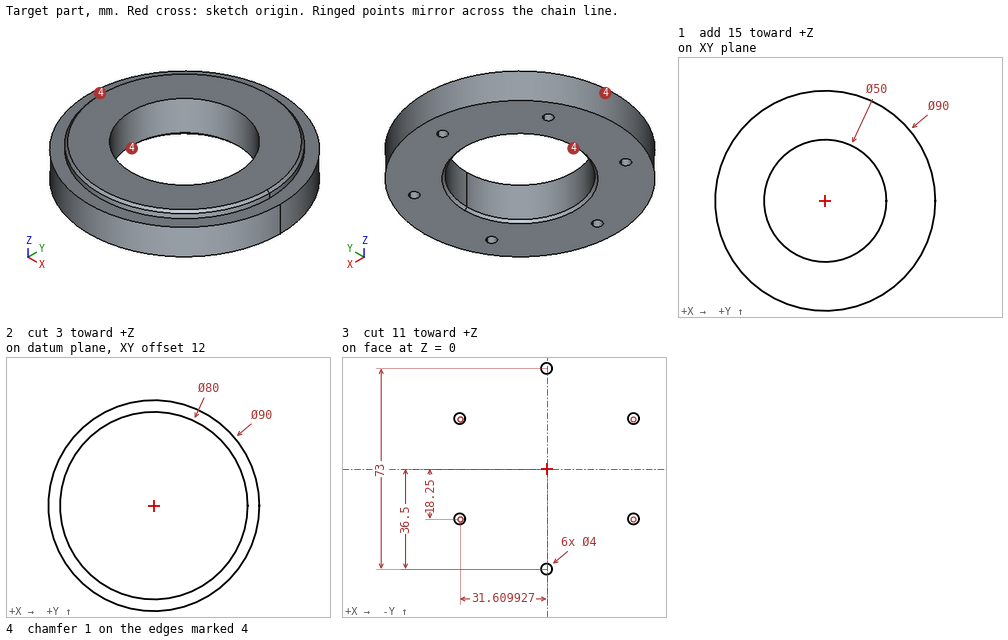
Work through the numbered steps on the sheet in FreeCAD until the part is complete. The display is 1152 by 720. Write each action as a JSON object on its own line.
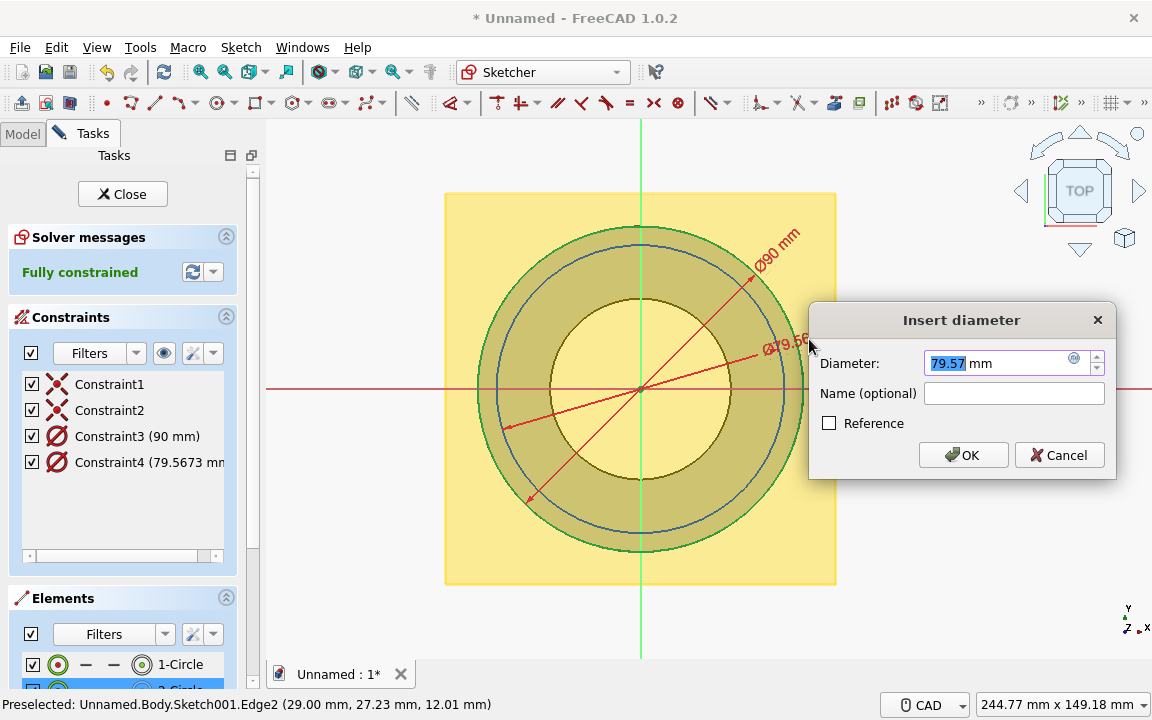
{"action": "type", "text": "80"}
{"action": "key", "text": "Return"}
{"action": "key", "text": "Escape"}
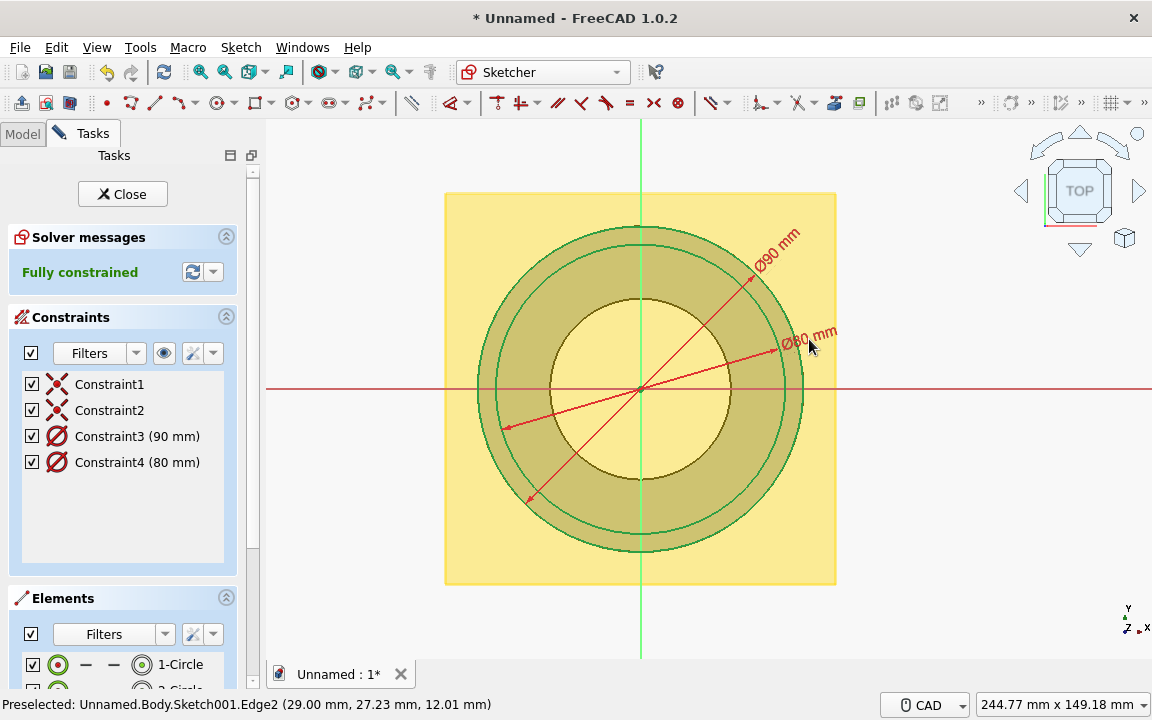
{"action": "left_click", "coordinate": [123, 194]}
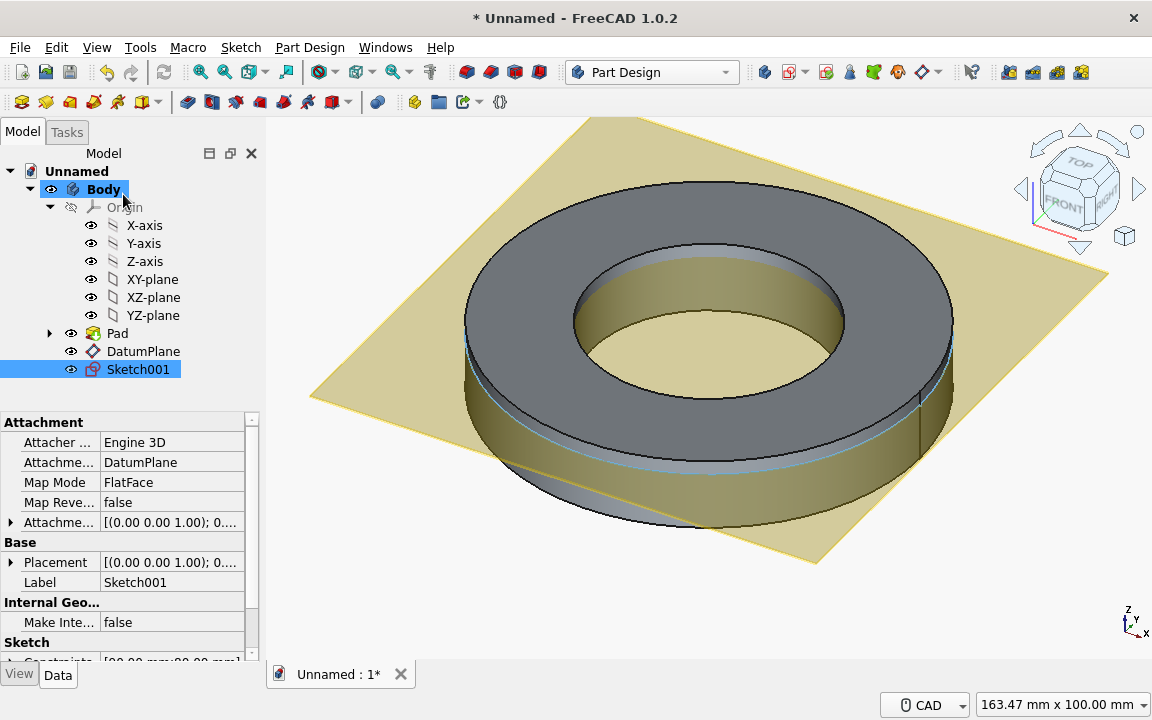
{"action": "left_click", "coordinate": [188, 102]}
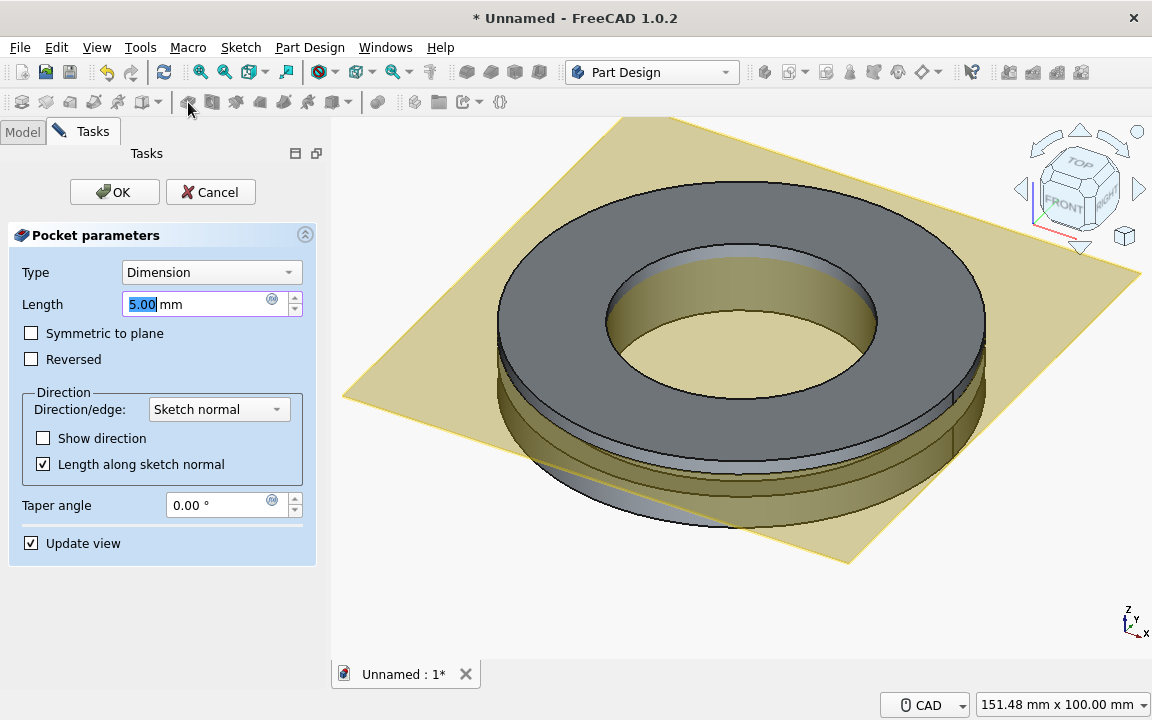
{"action": "type", "text": "3"}
{"action": "key", "text": "Tab"}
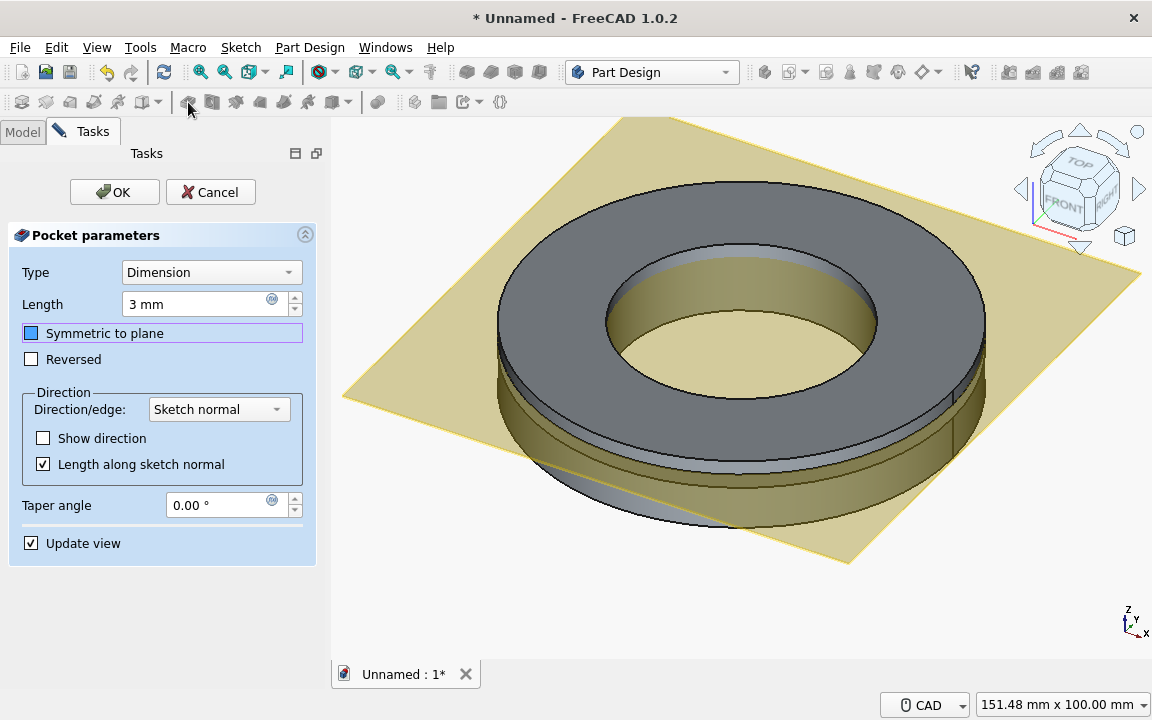
{"action": "left_click", "coordinate": [30, 359]}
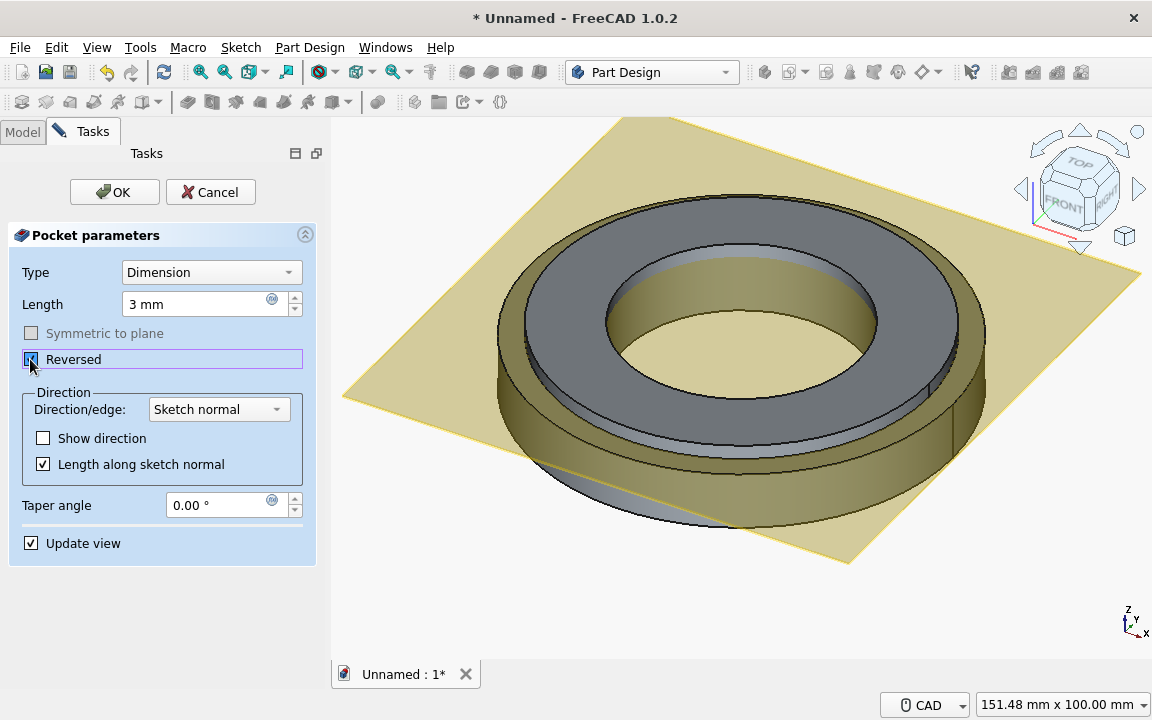
{"action": "left_click", "coordinate": [115, 192]}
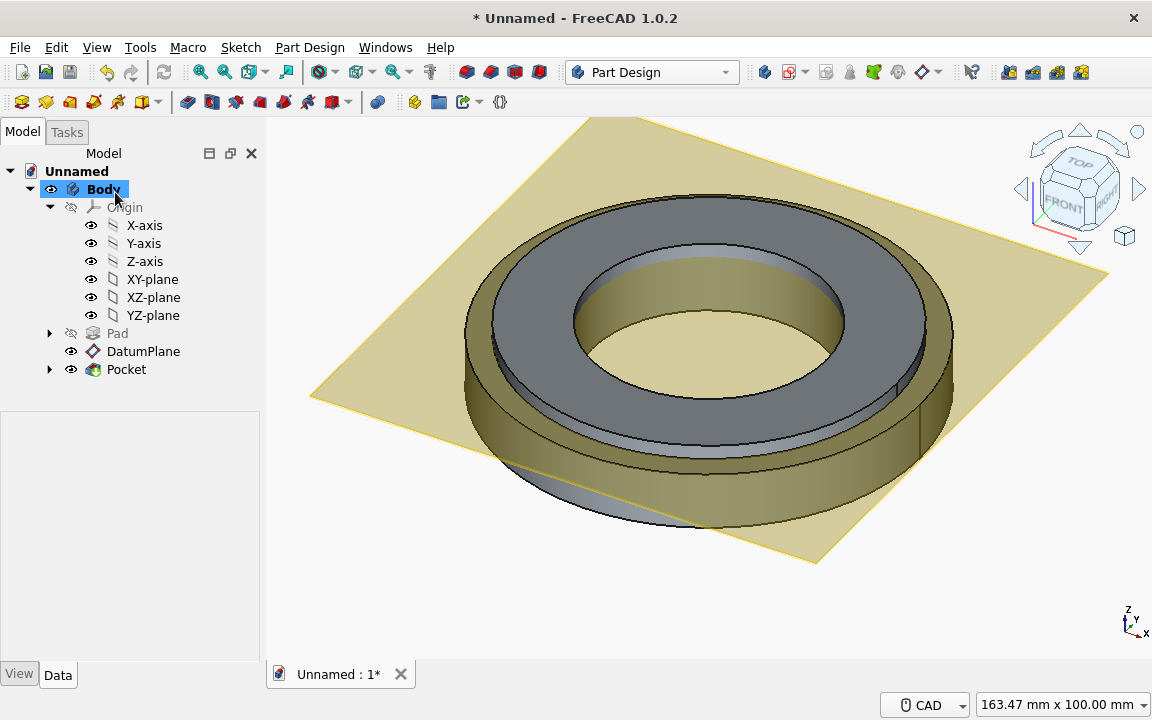
{"action": "left_click", "coordinate": [116, 351]}
{"action": "key", "text": "space"}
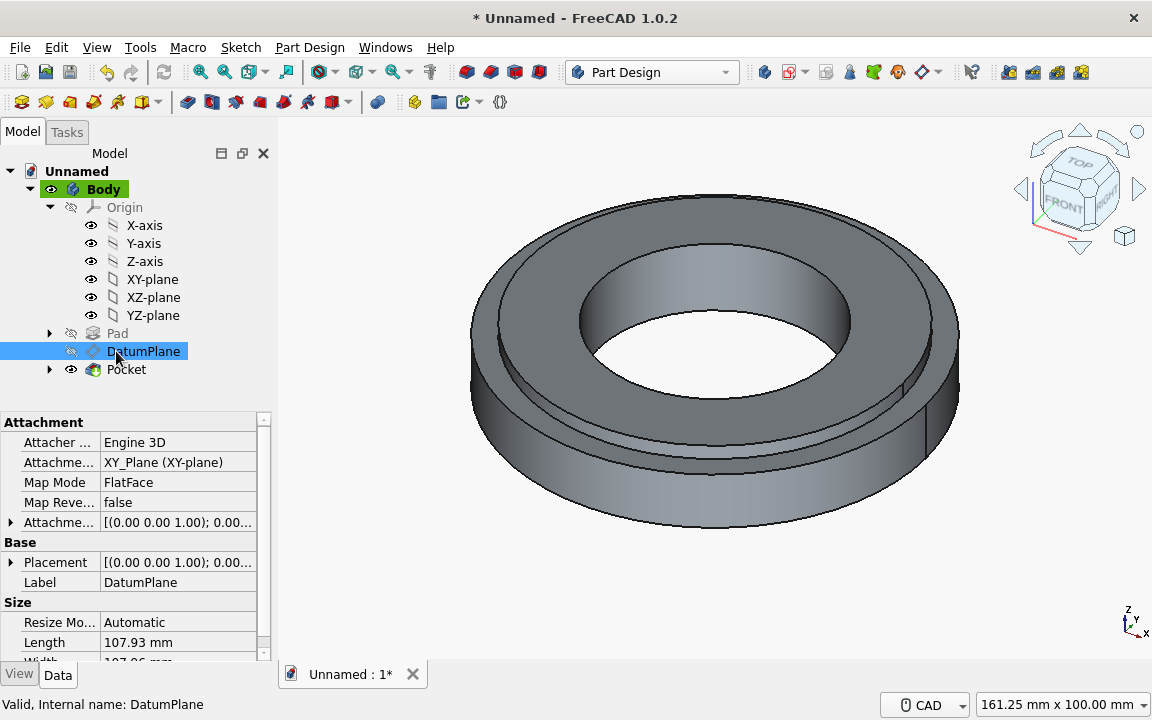
{"action": "key", "text": "5"}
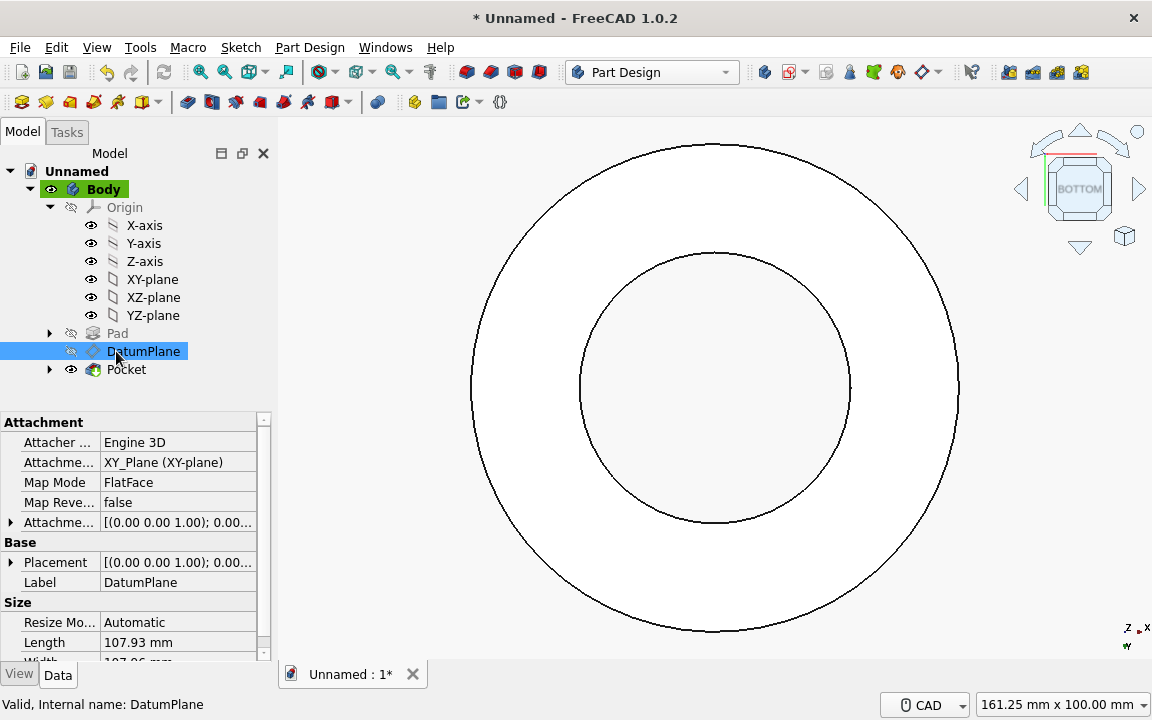
{"action": "left_click", "coordinate": [854, 526]}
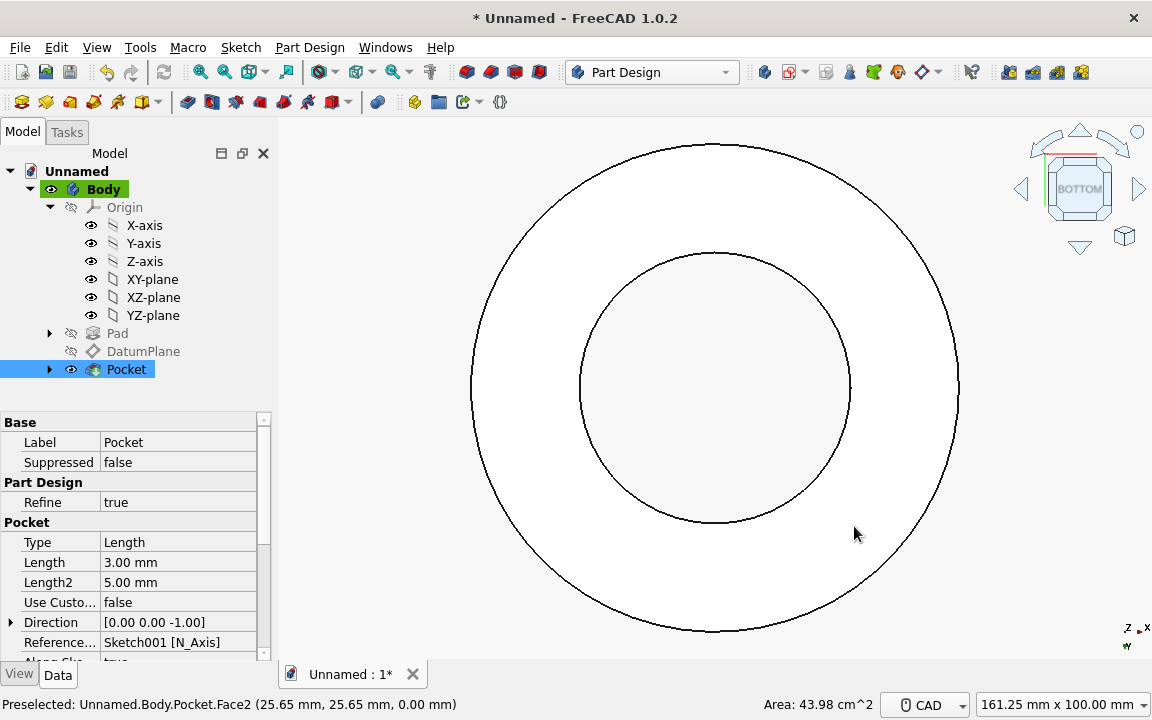
{"action": "left_click", "coordinate": [790, 72]}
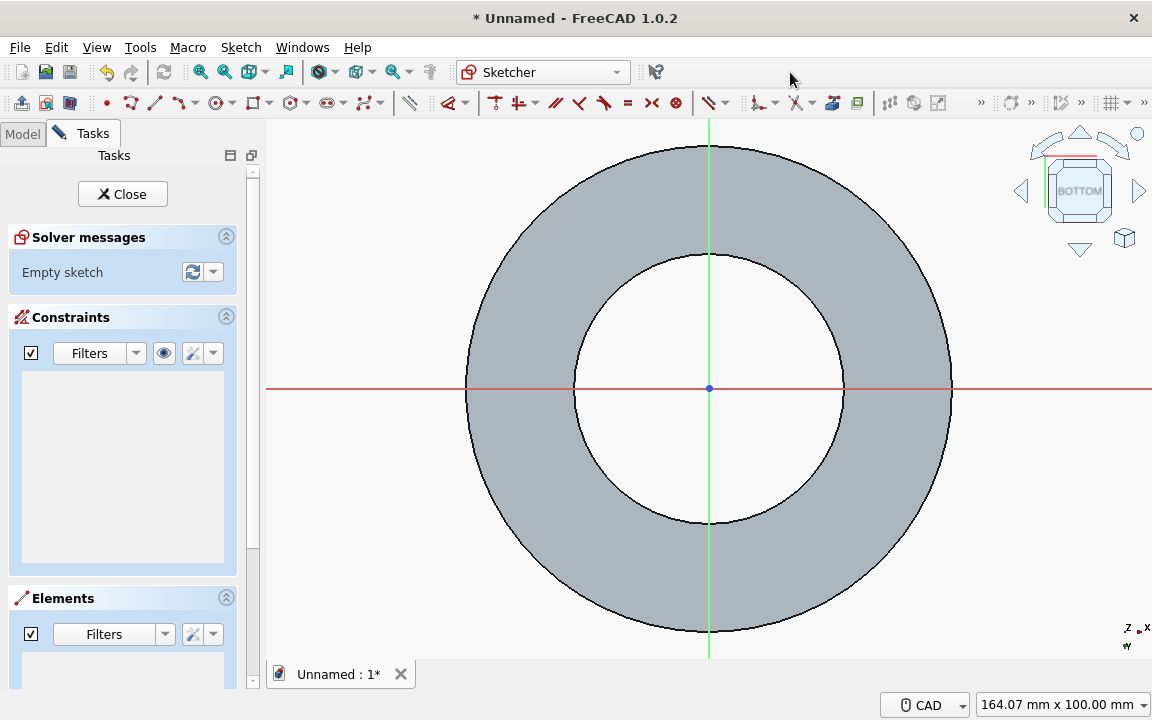
{"action": "key", "text": "g c"}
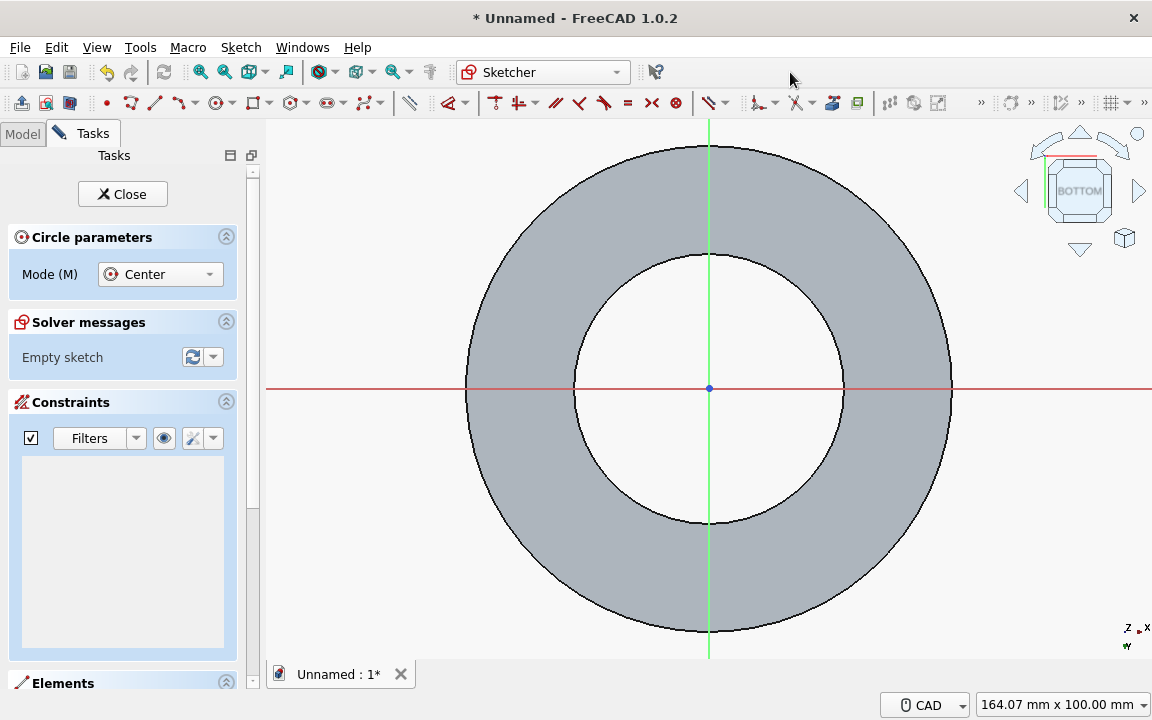
{"action": "scroll", "coordinate": [709, 586], "scroll_direction": "up", "scroll_amount": 4}